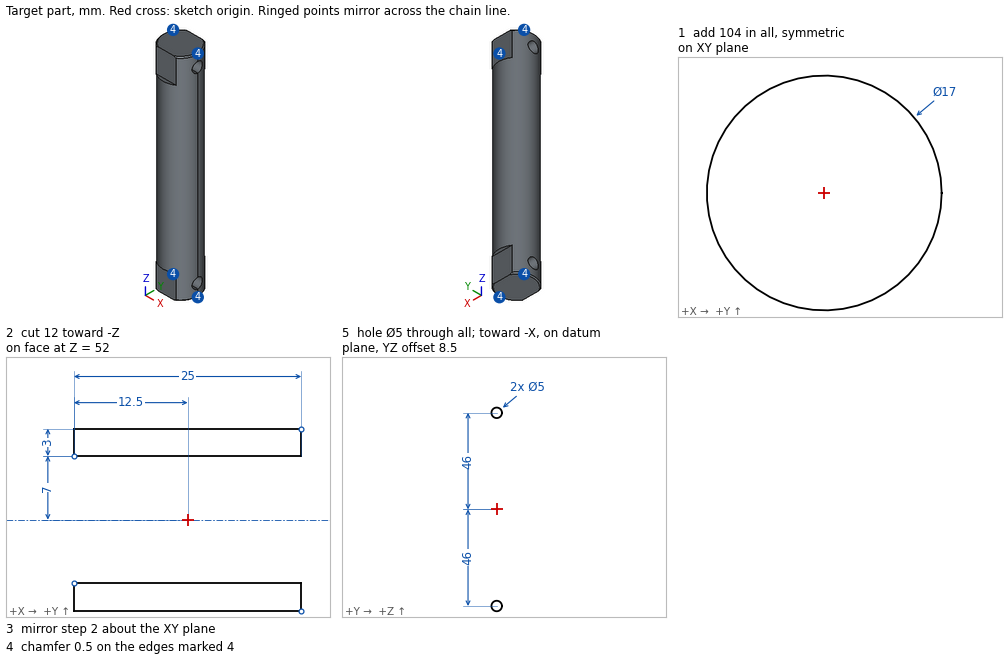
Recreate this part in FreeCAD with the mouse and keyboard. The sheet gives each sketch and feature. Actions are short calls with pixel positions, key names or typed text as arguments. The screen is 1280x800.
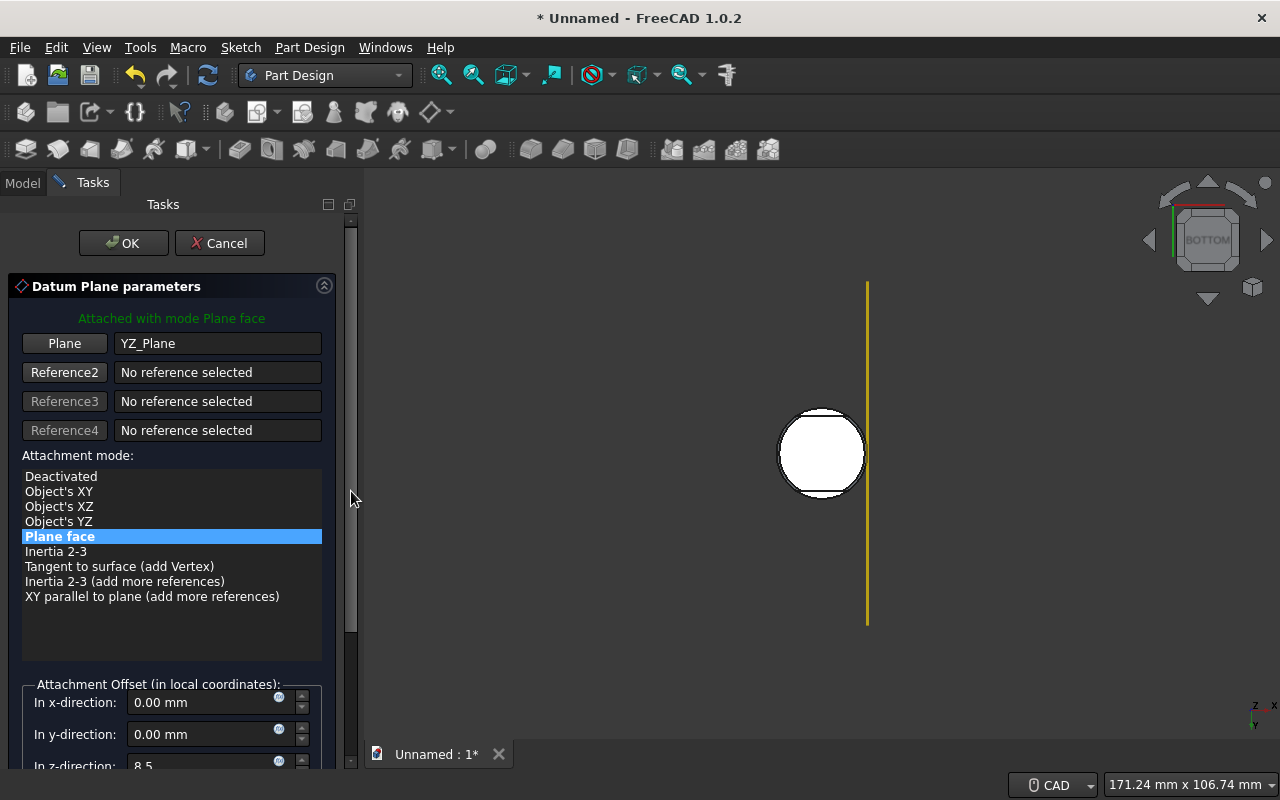
click(124, 243)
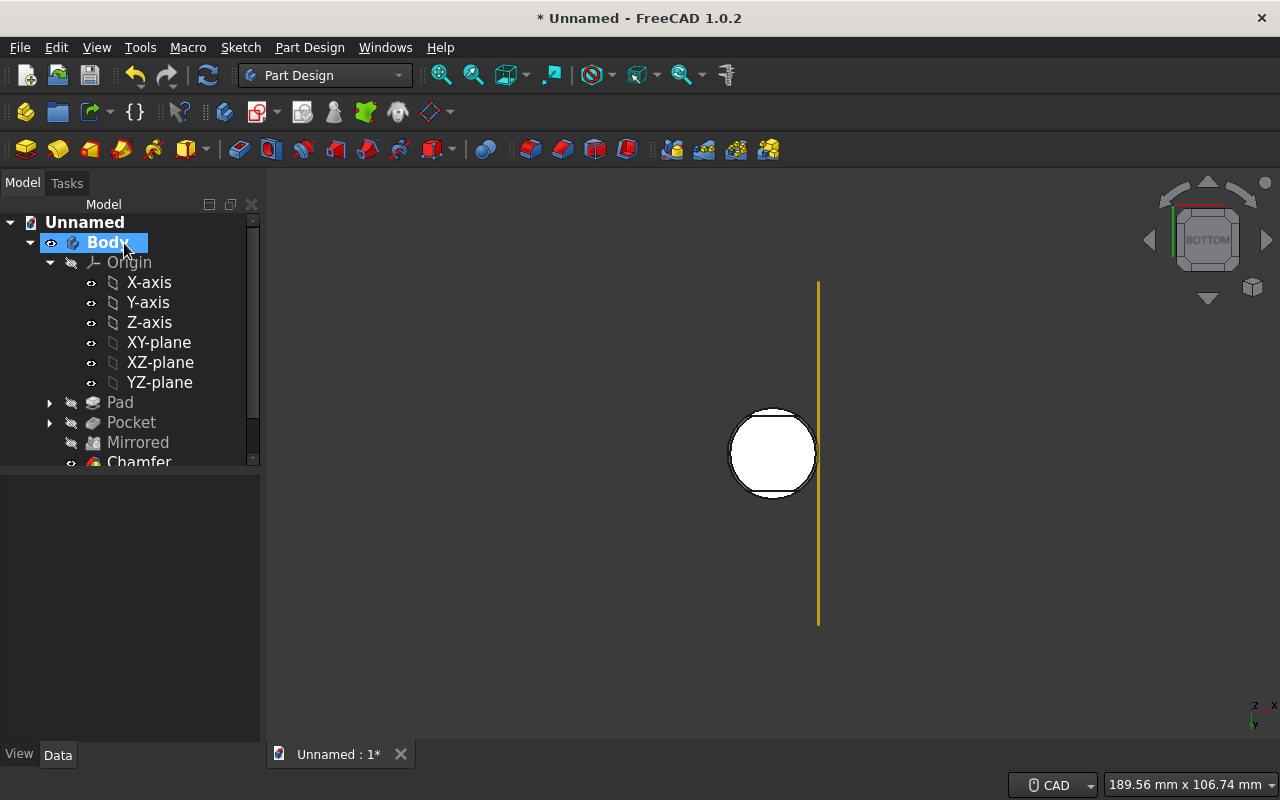
scroll(100, 338, down, 3)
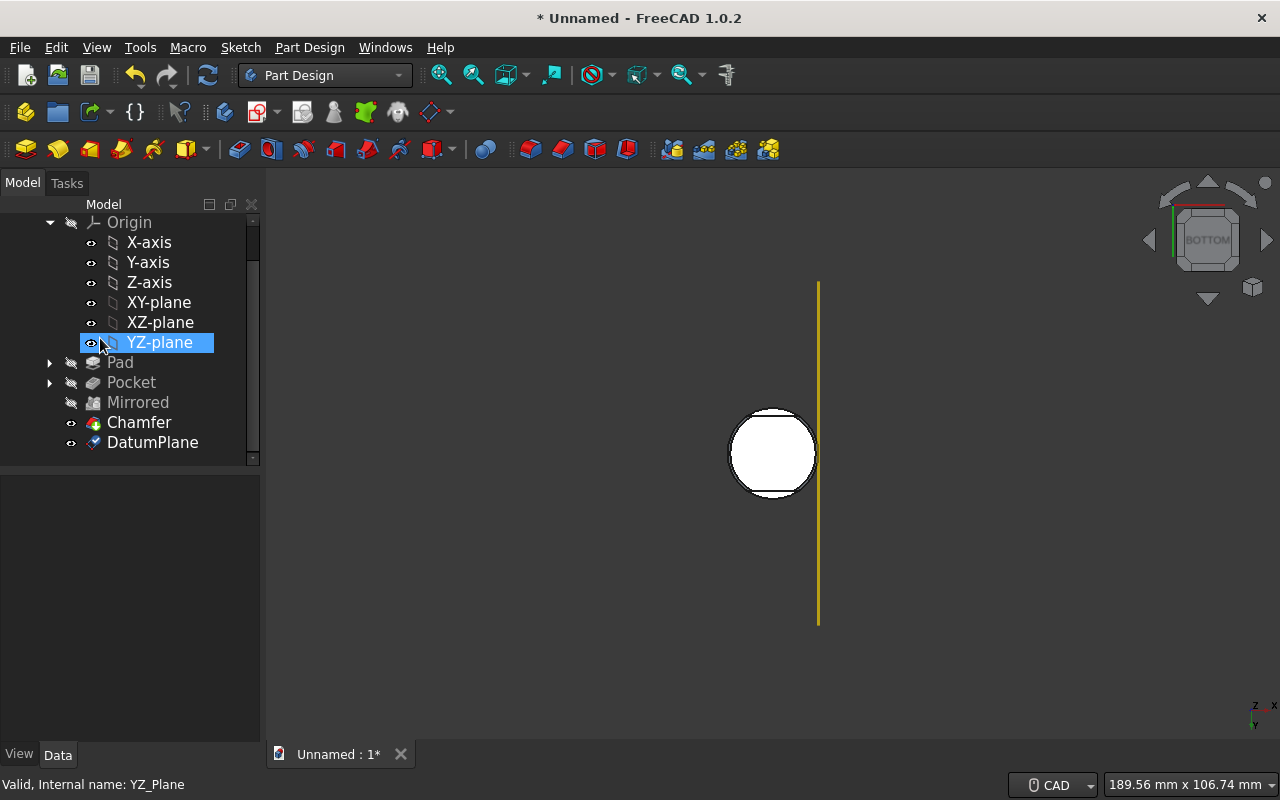
click(116, 443)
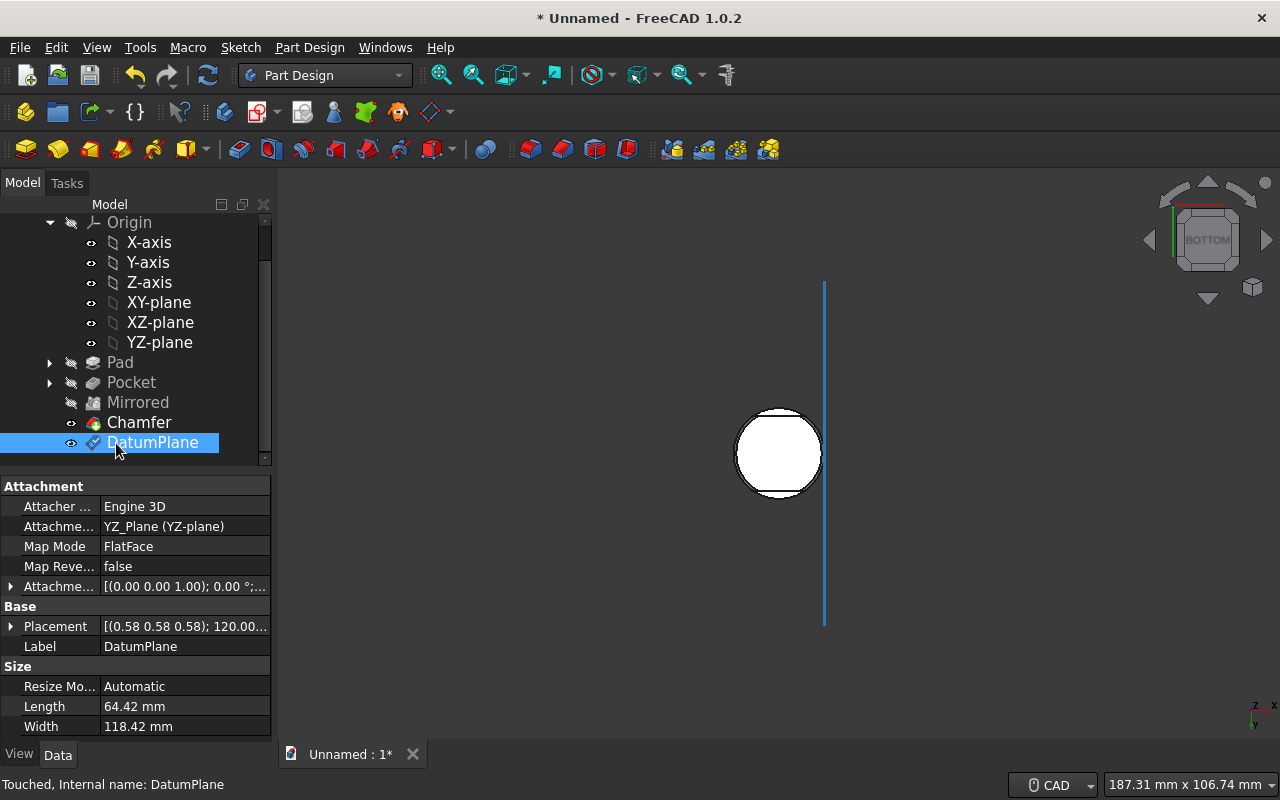
click(258, 112)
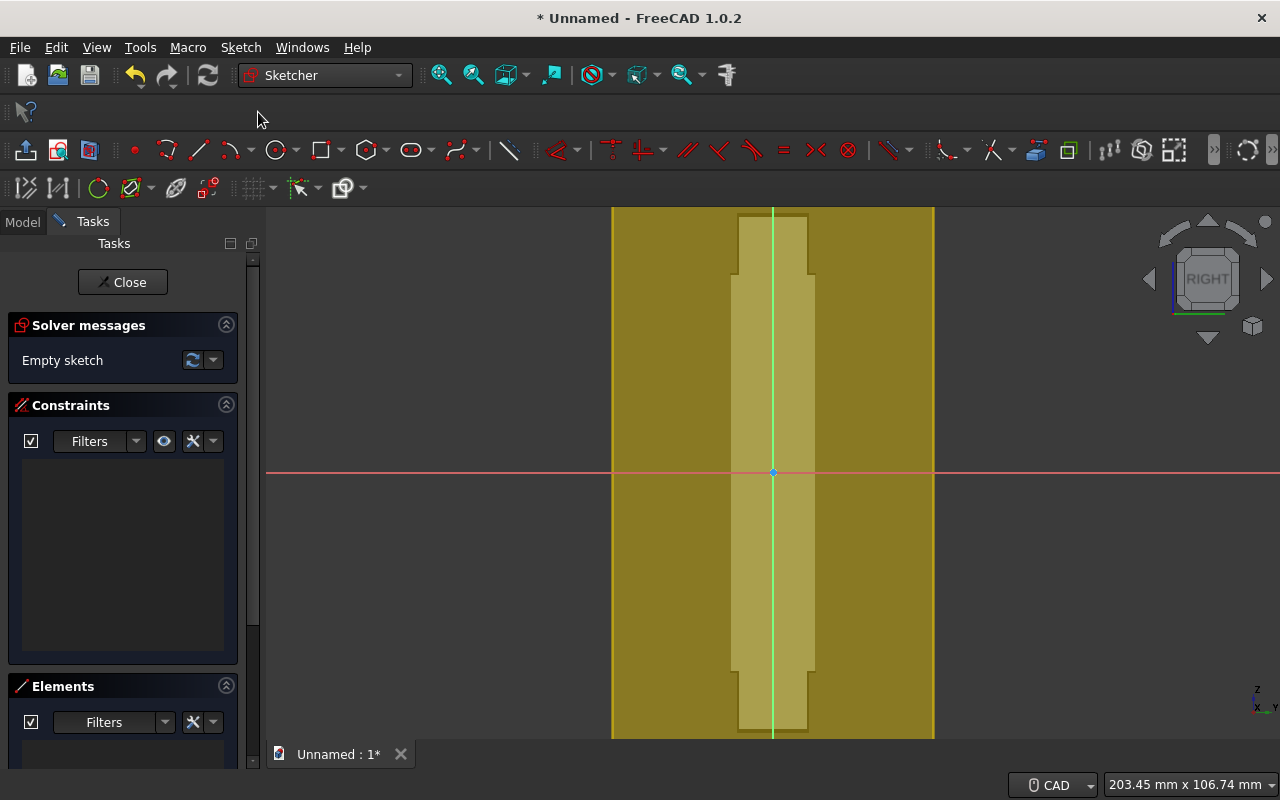
scroll(565, 473, down, 2)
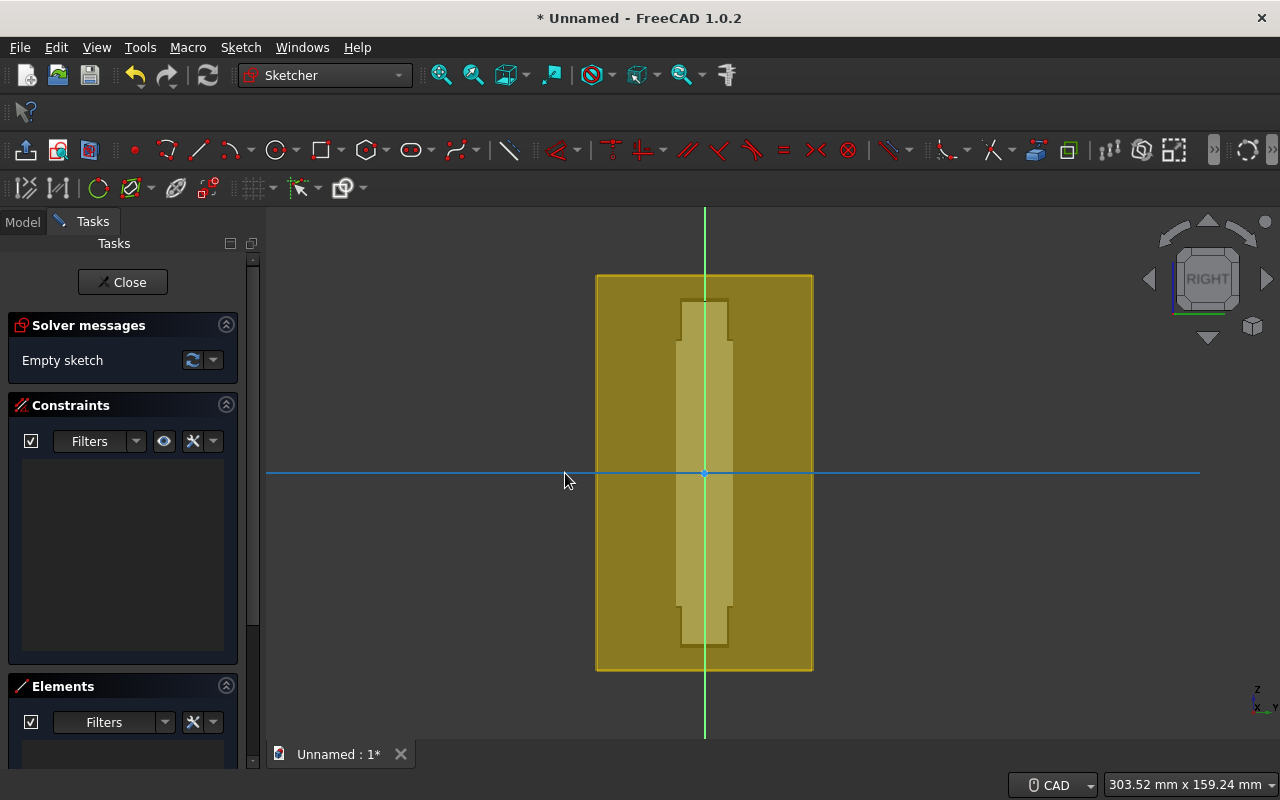
click(276, 150)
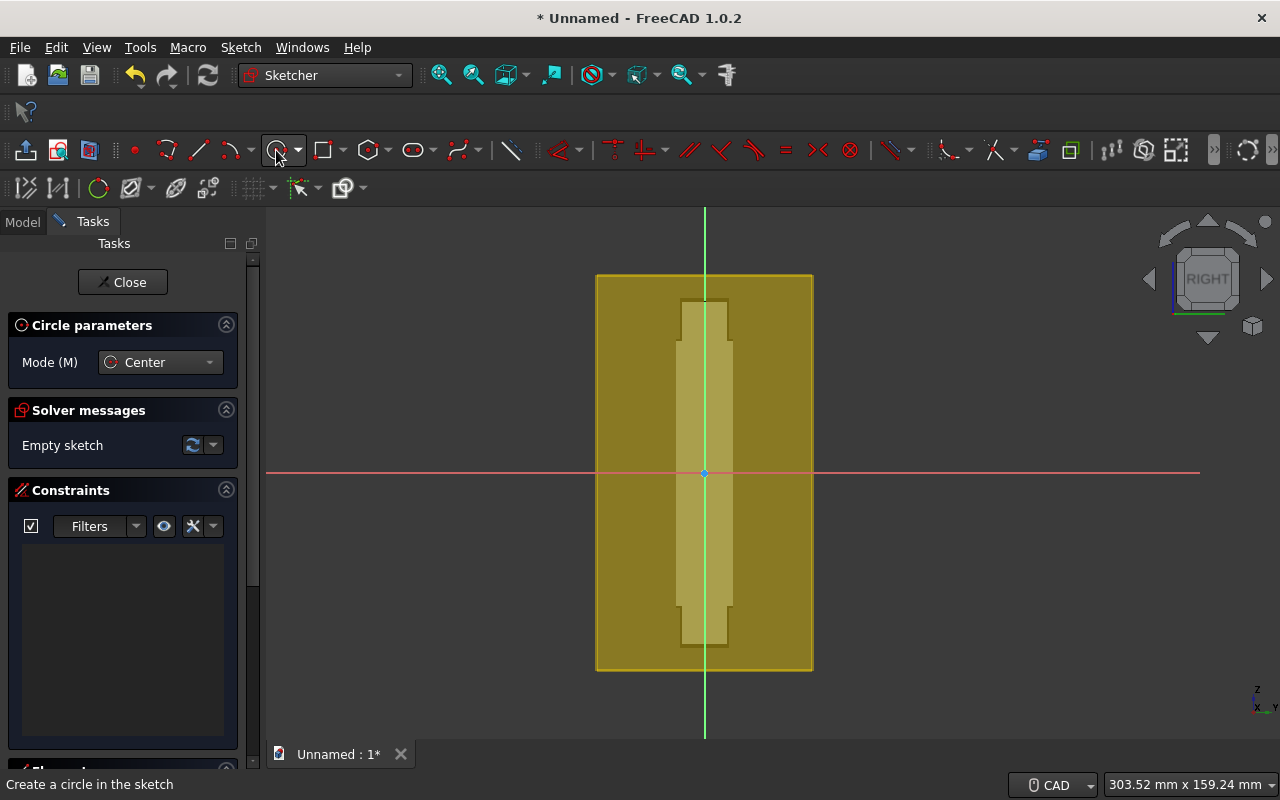
scroll(705, 319, up, 5)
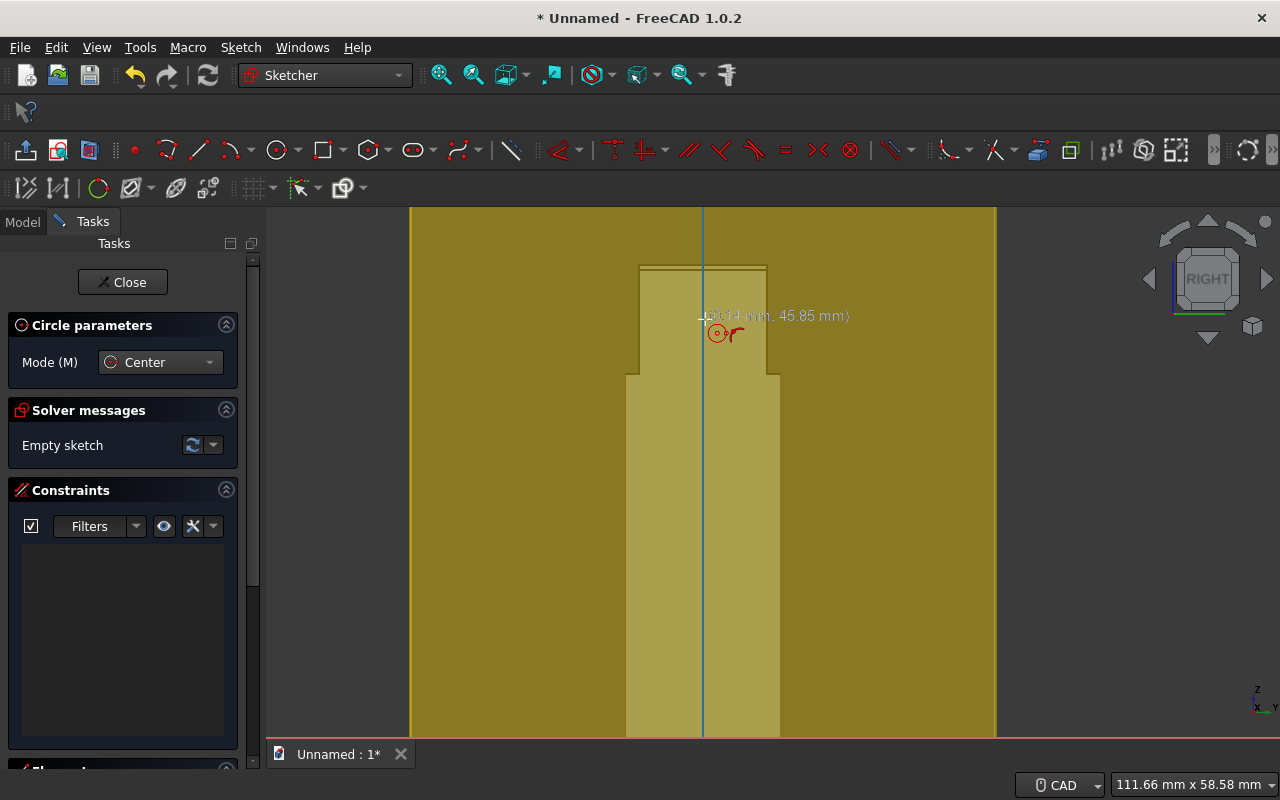
click(703, 320)
click(719, 304)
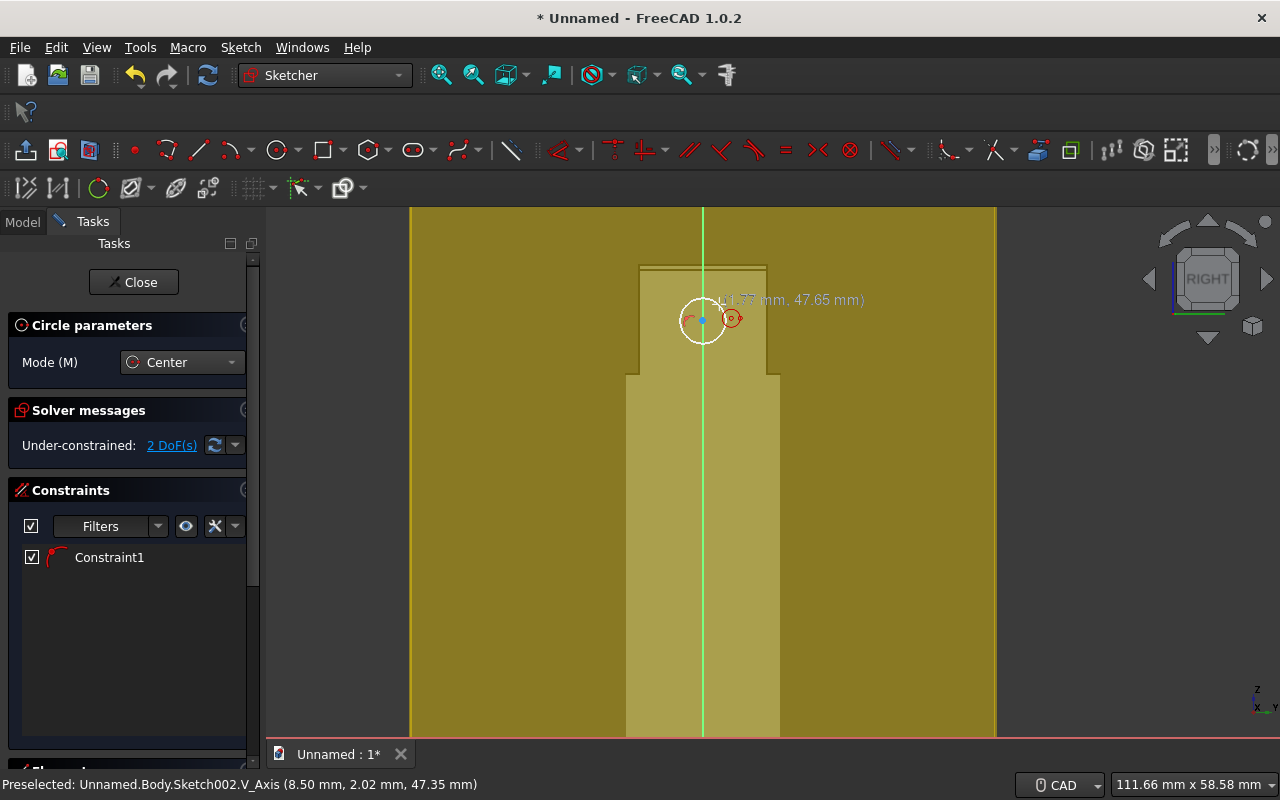
scroll(705, 319, down, 5)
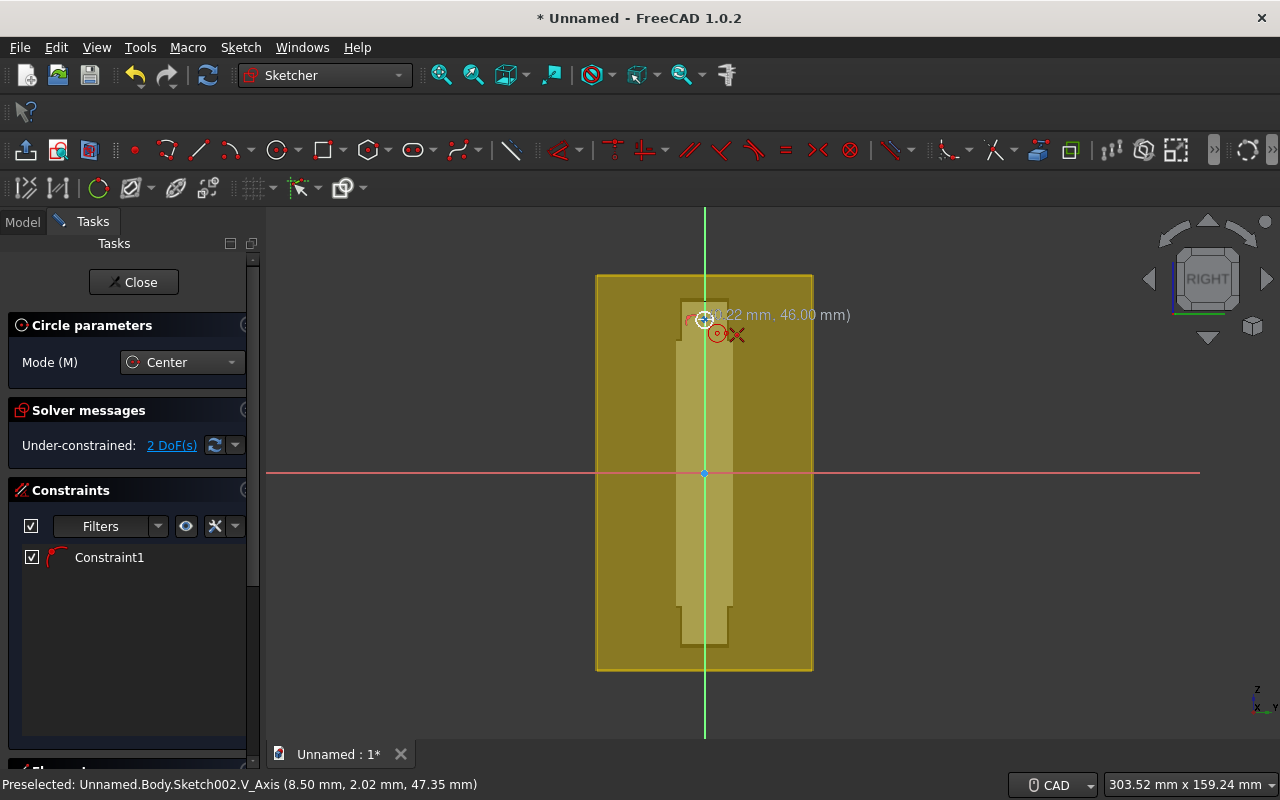
scroll(705, 627, up, 5)